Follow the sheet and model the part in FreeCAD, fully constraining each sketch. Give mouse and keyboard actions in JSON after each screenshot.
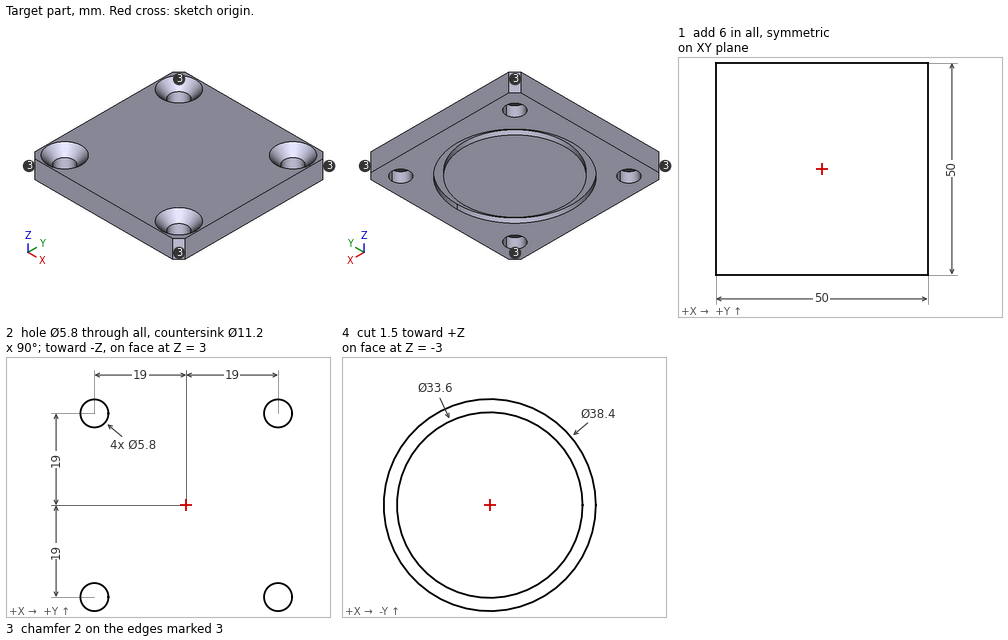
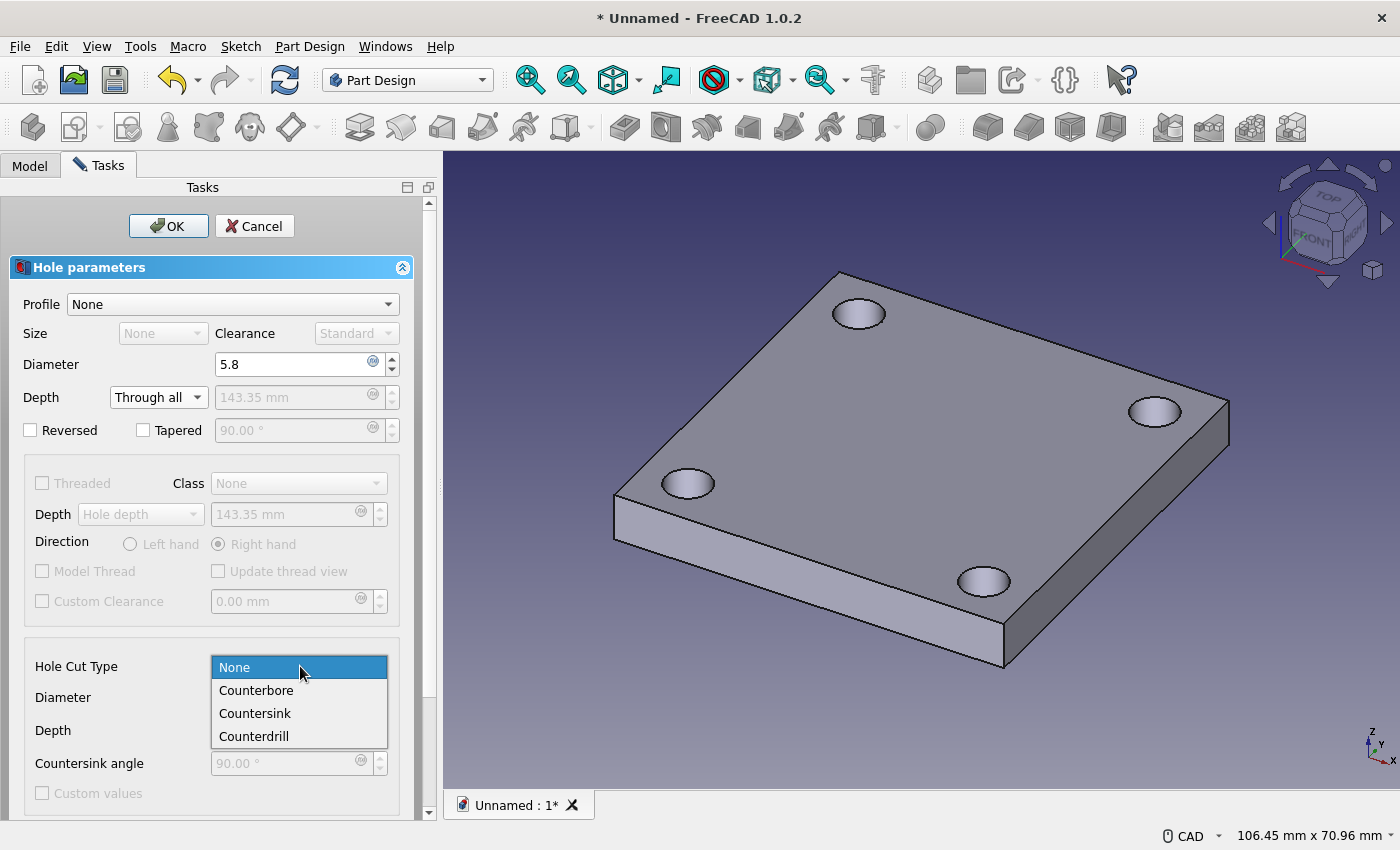
{"action": "left_click", "coordinate": [298, 714]}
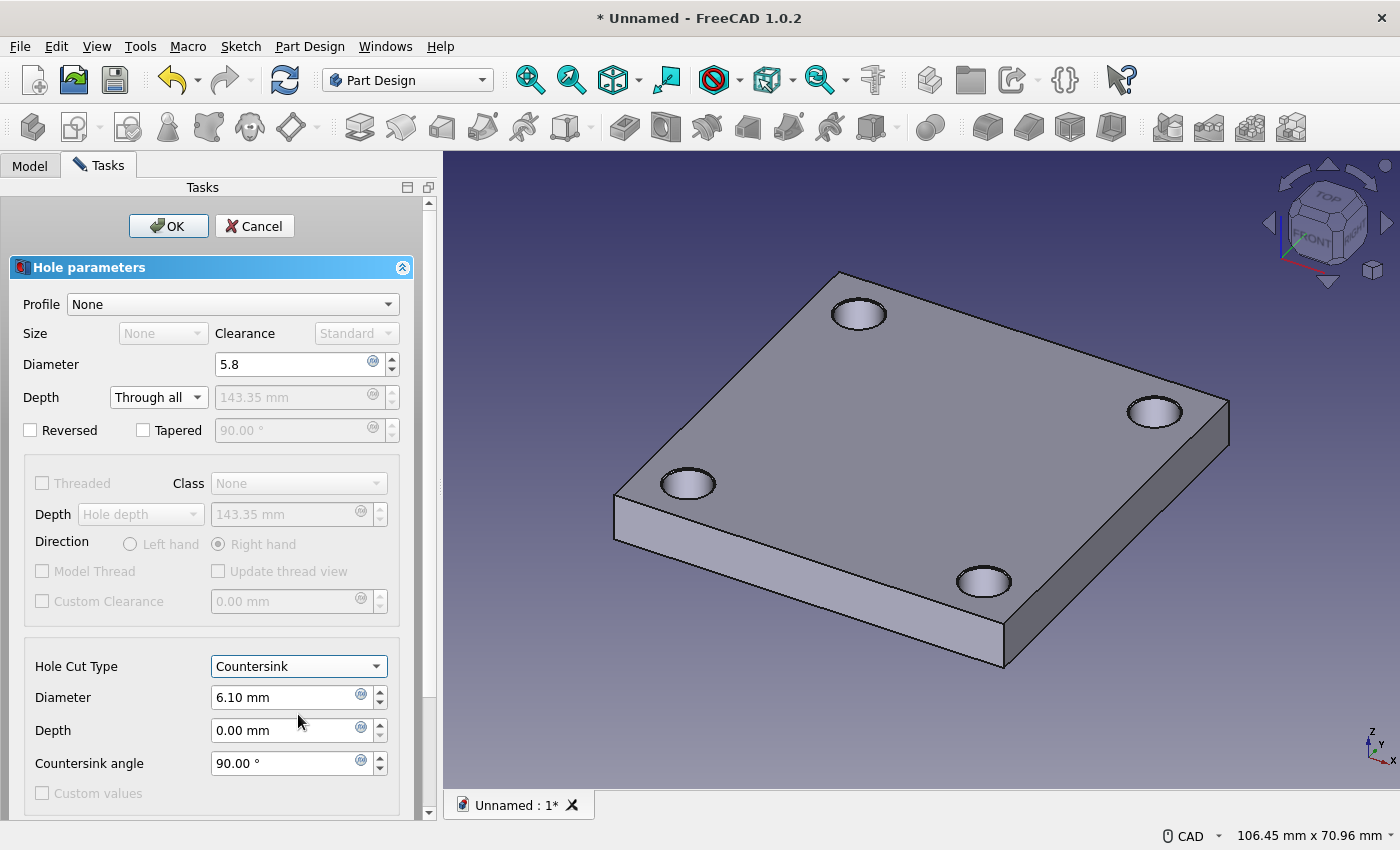
{"action": "triple_click", "coordinate": [292, 698]}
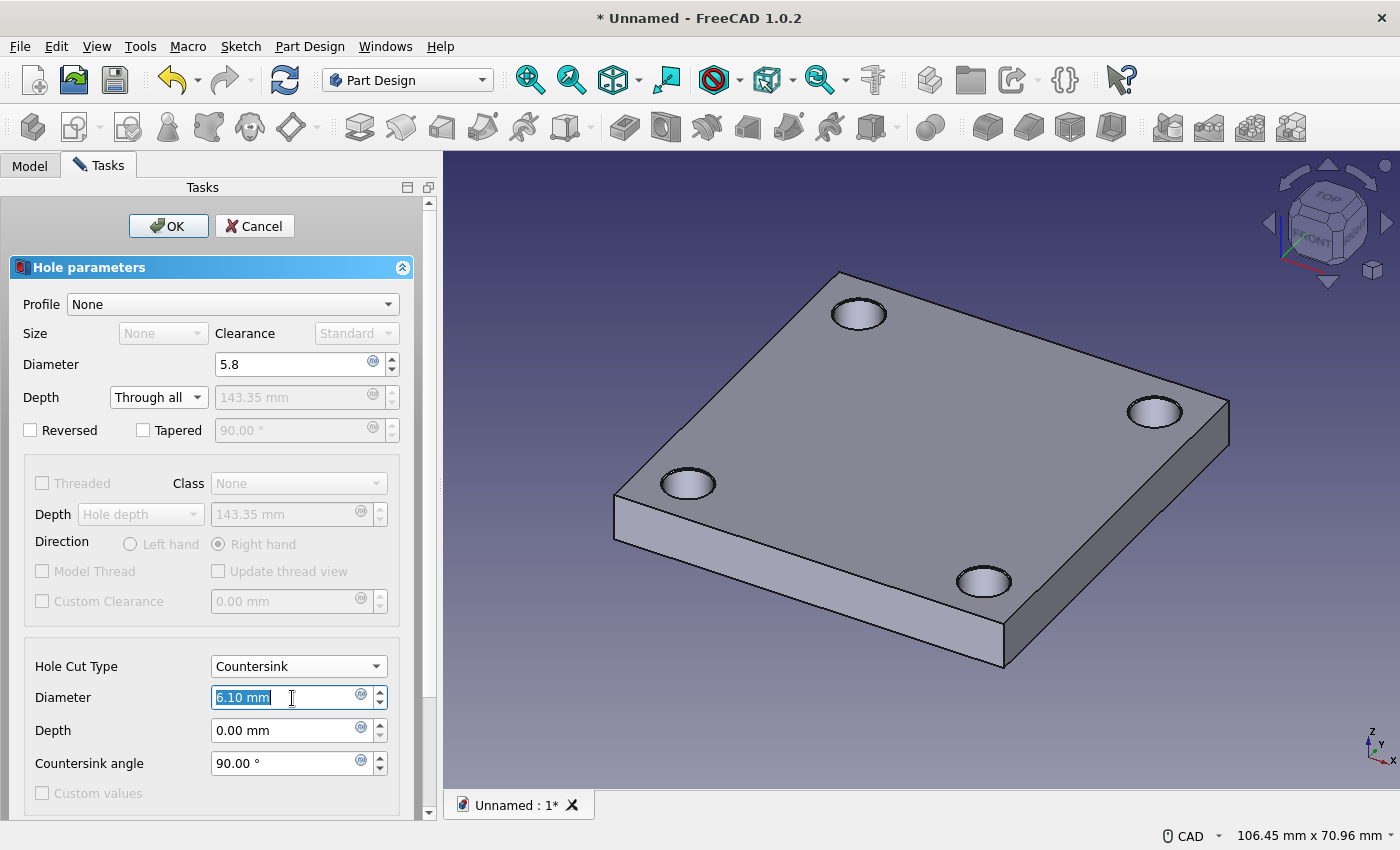
{"action": "type", "text": "11.2"}
{"action": "key", "text": "Tab"}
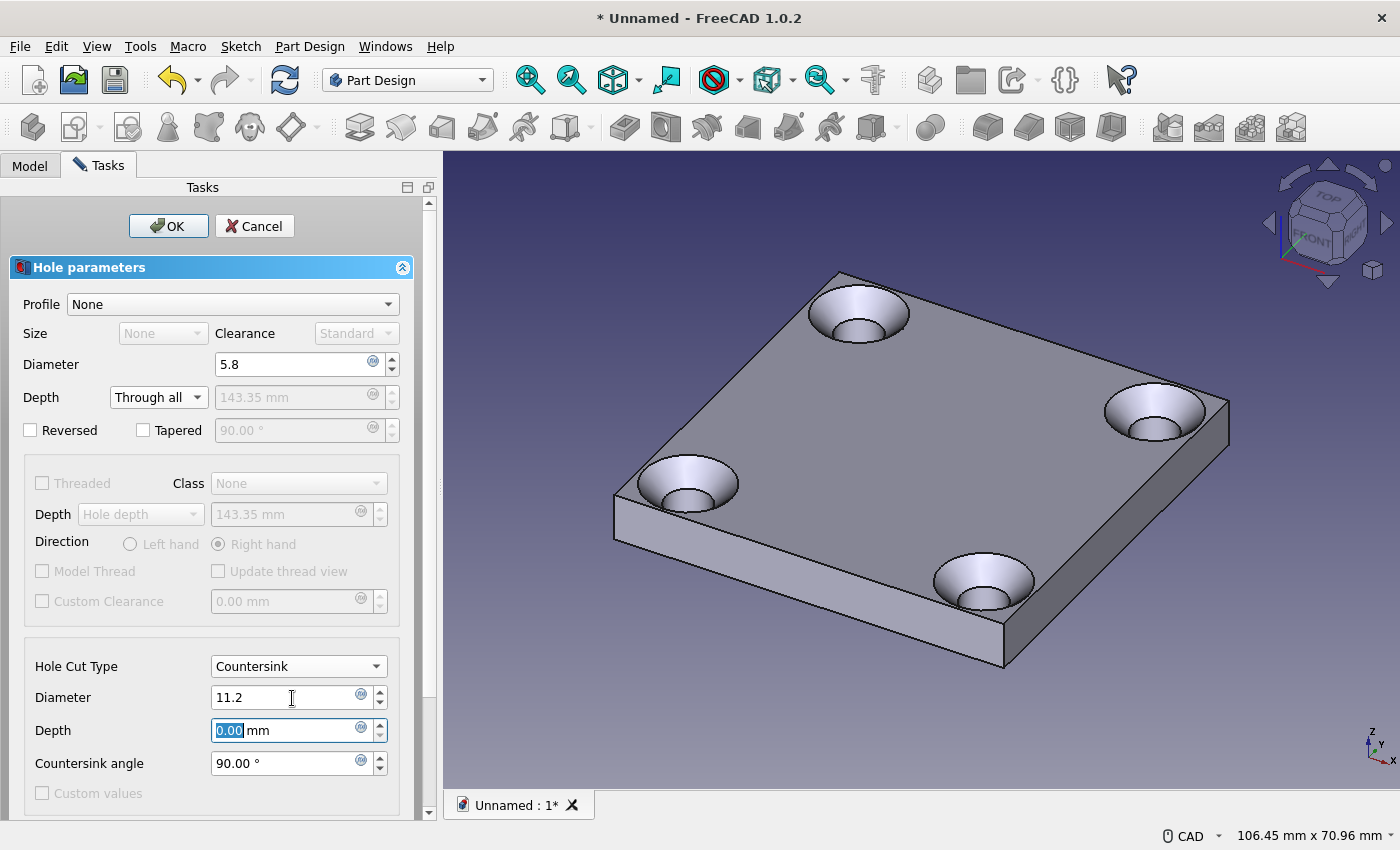
{"action": "left_click", "coordinate": [169, 226]}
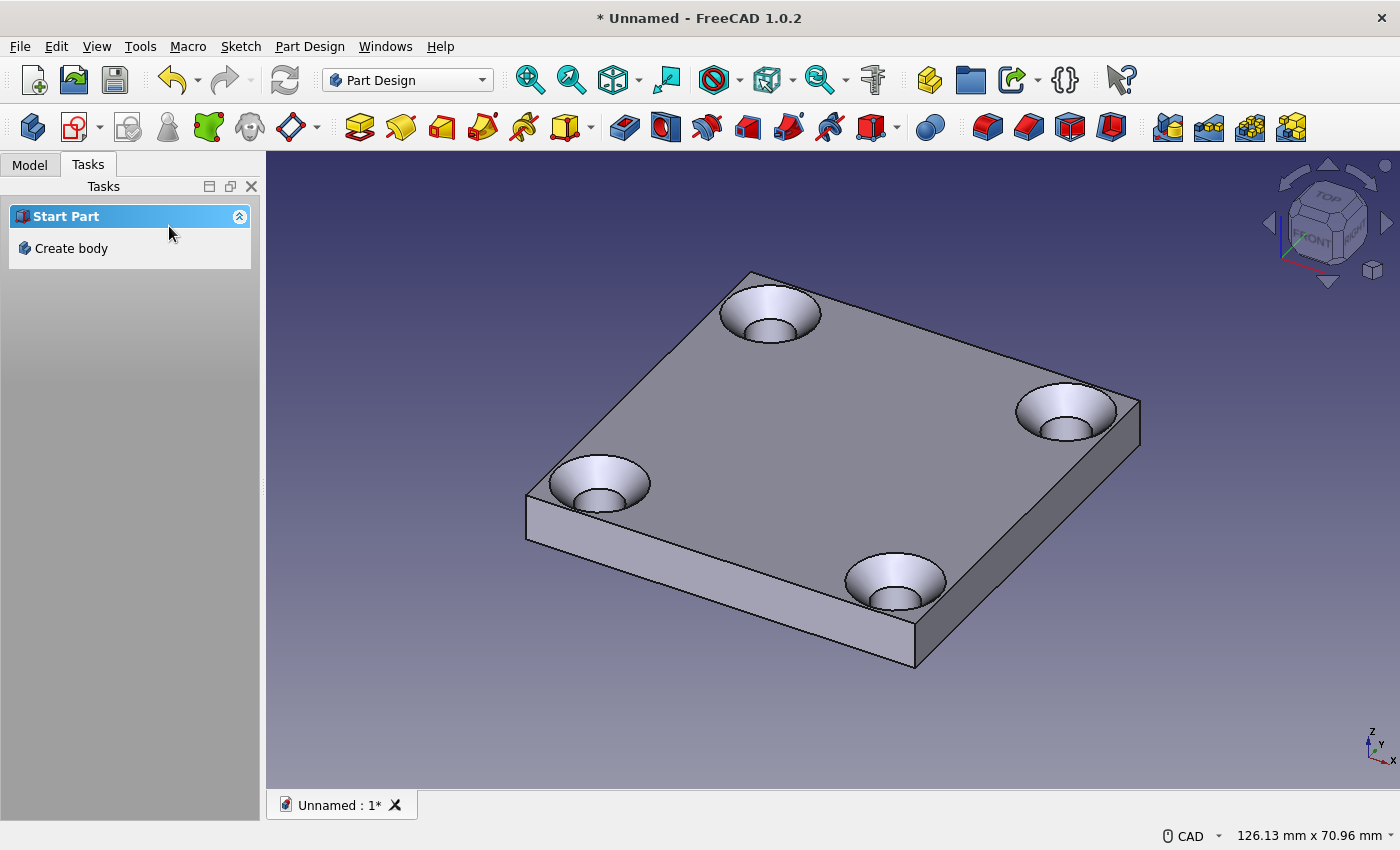
{"action": "left_click", "coordinate": [915, 645]}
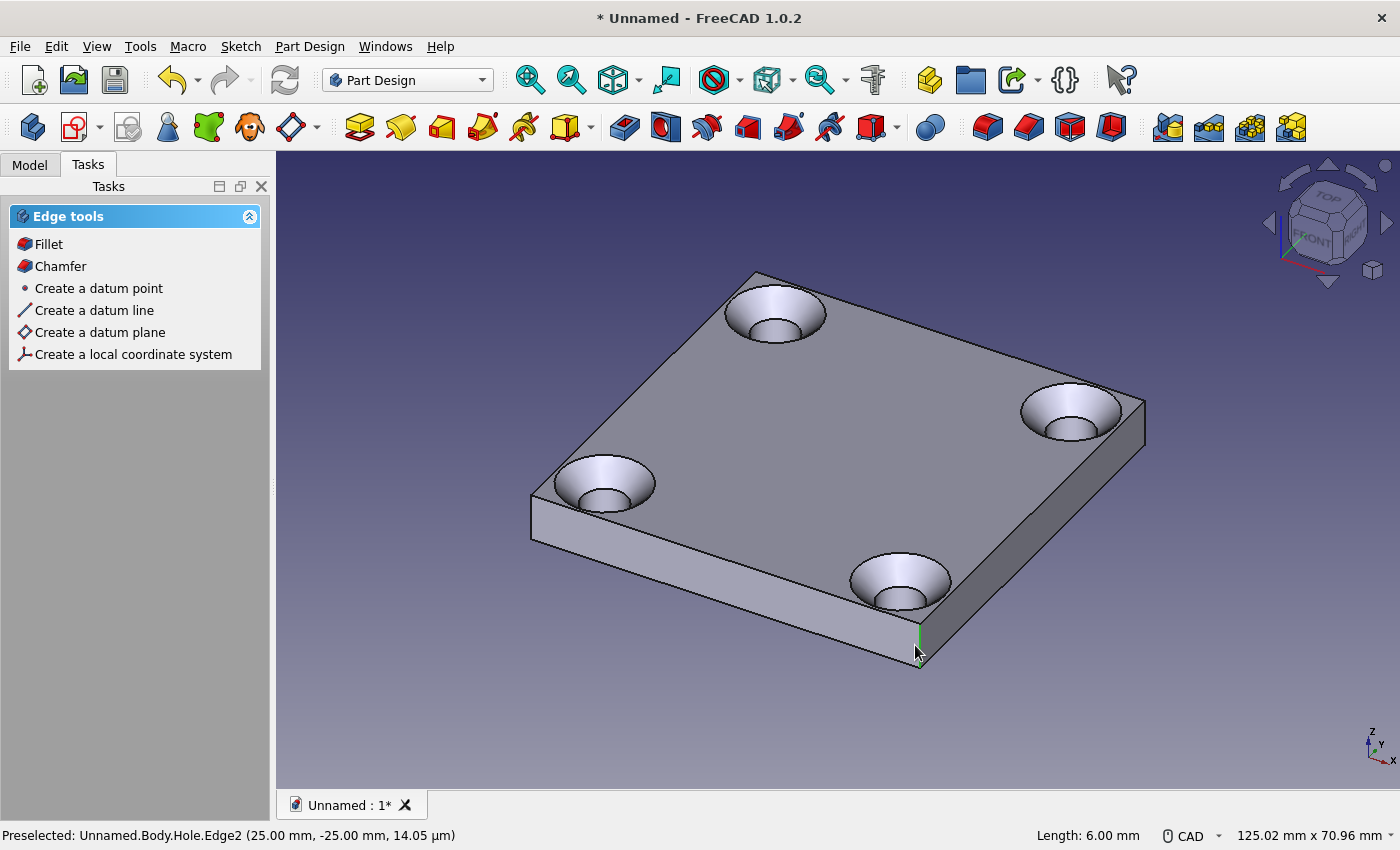
{"action": "key", "text": "0"}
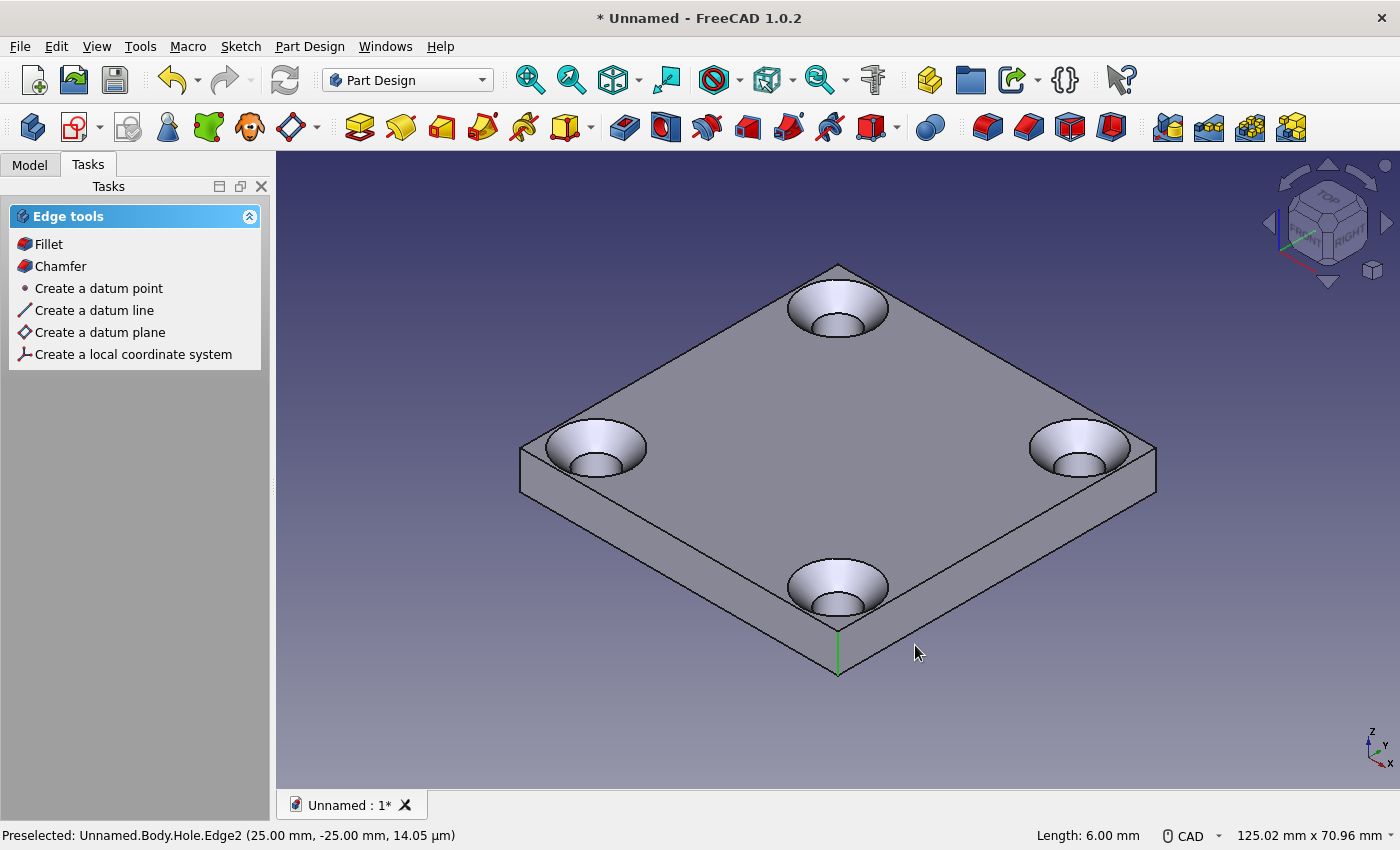
{"action": "key", "text": "2"}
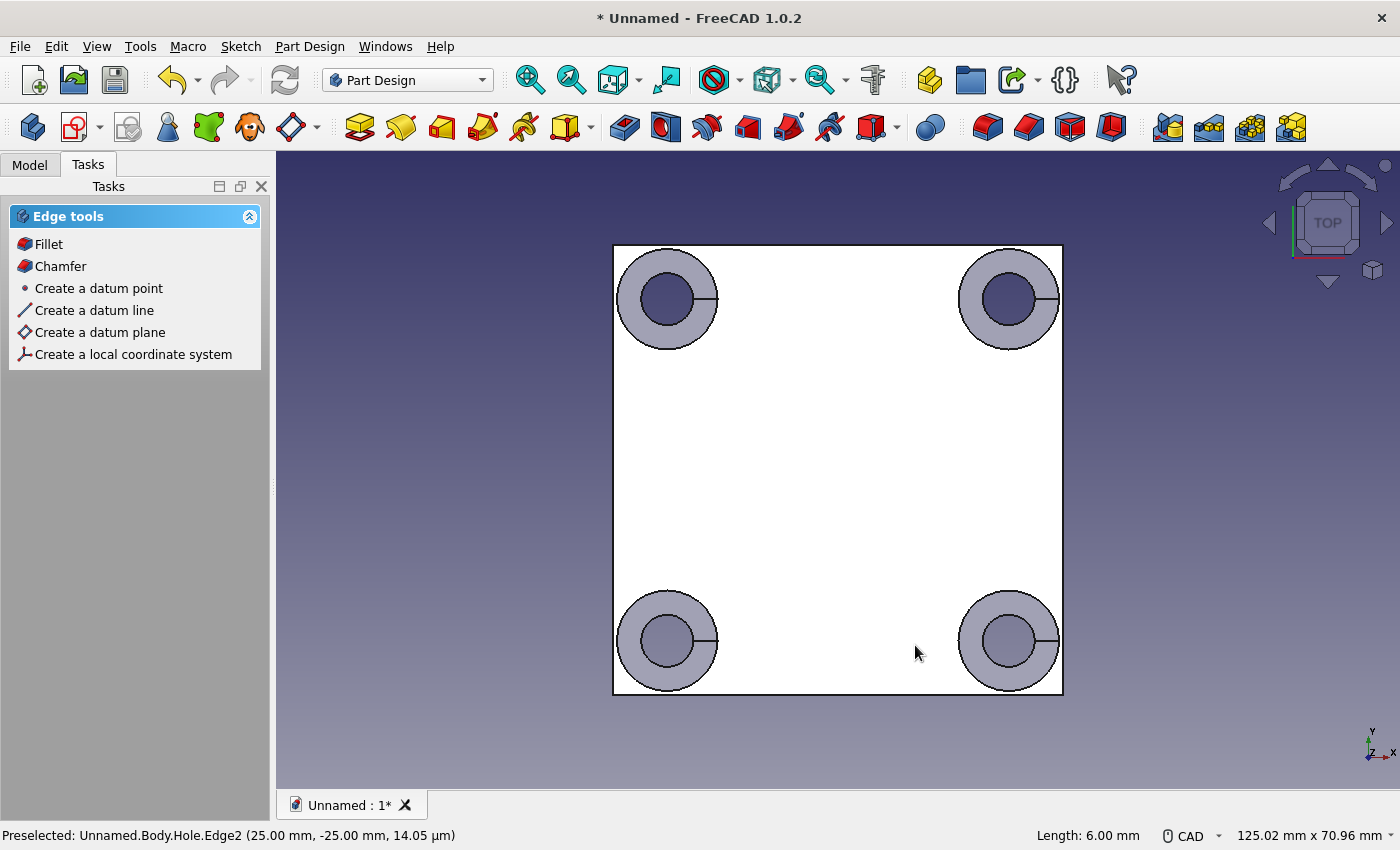
{"action": "key", "text": "1"}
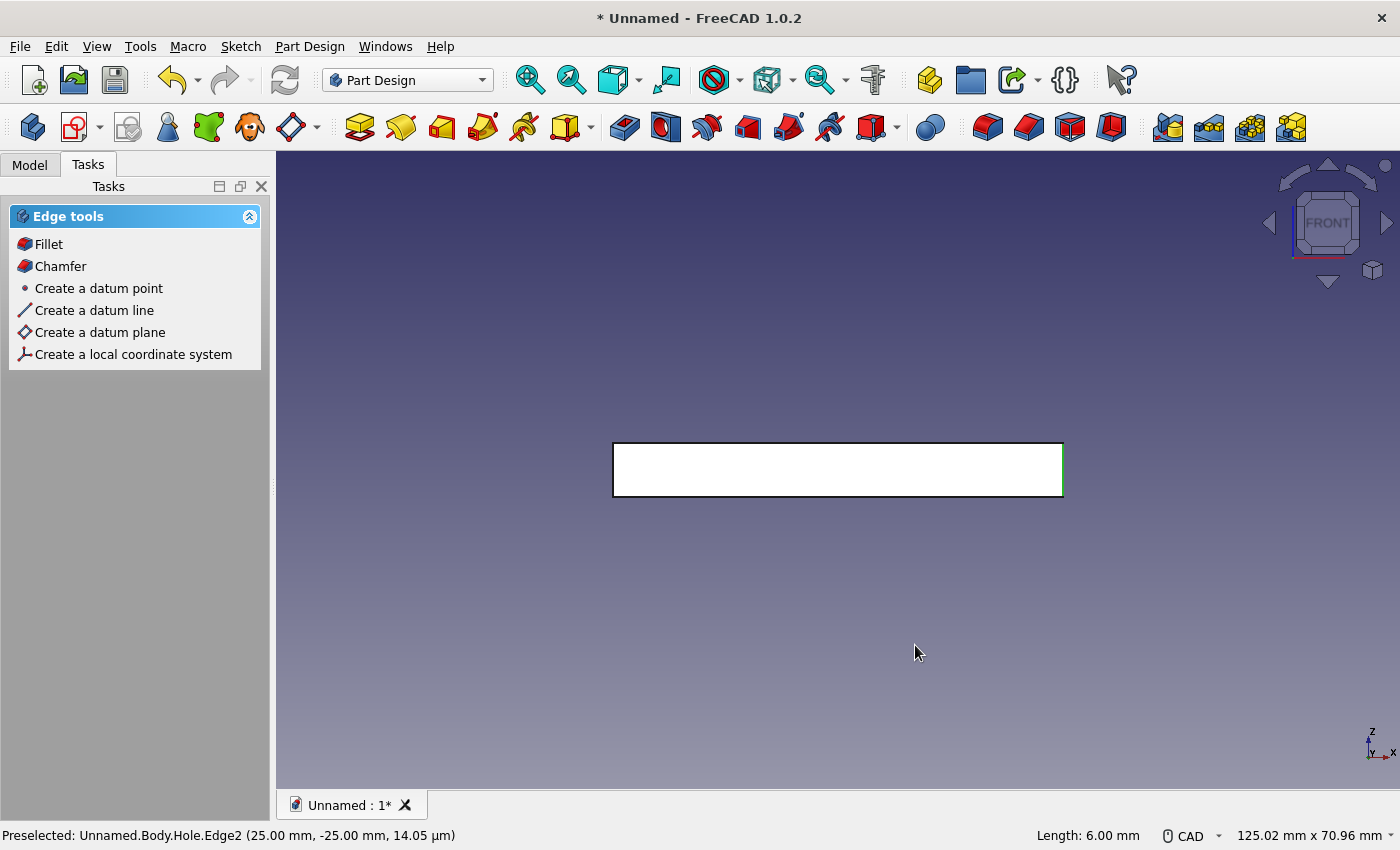
{"action": "left_click", "coordinate": [531, 80]}